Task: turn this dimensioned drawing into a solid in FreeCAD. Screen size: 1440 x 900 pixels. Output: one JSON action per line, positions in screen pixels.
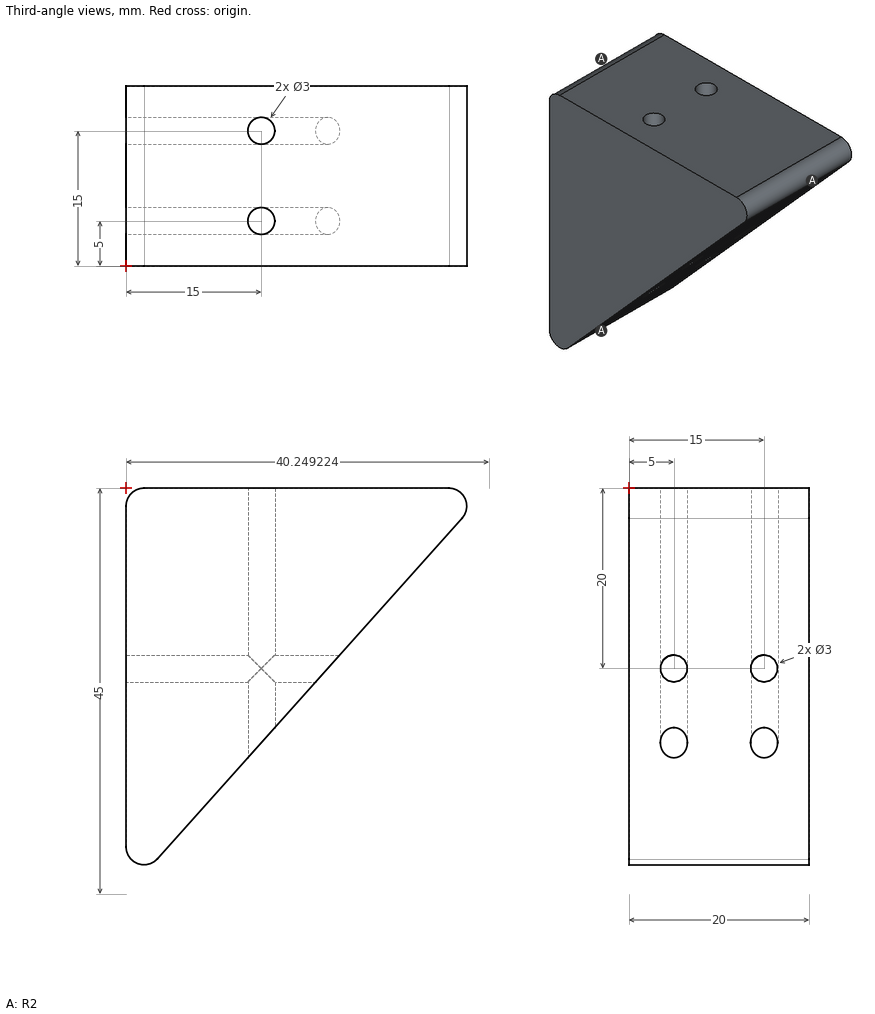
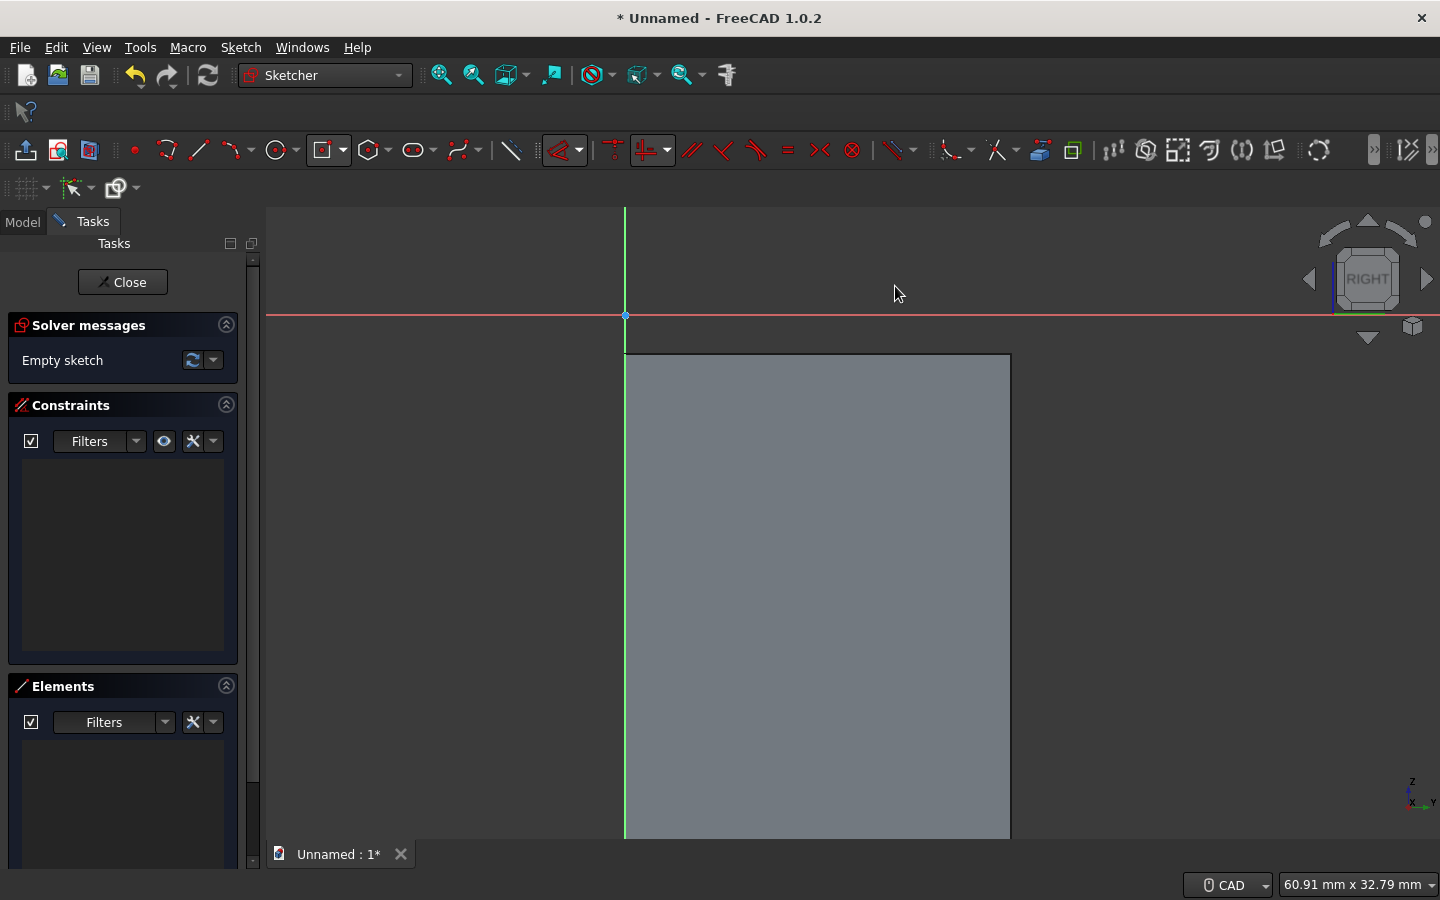
{"action": "key", "text": "g c"}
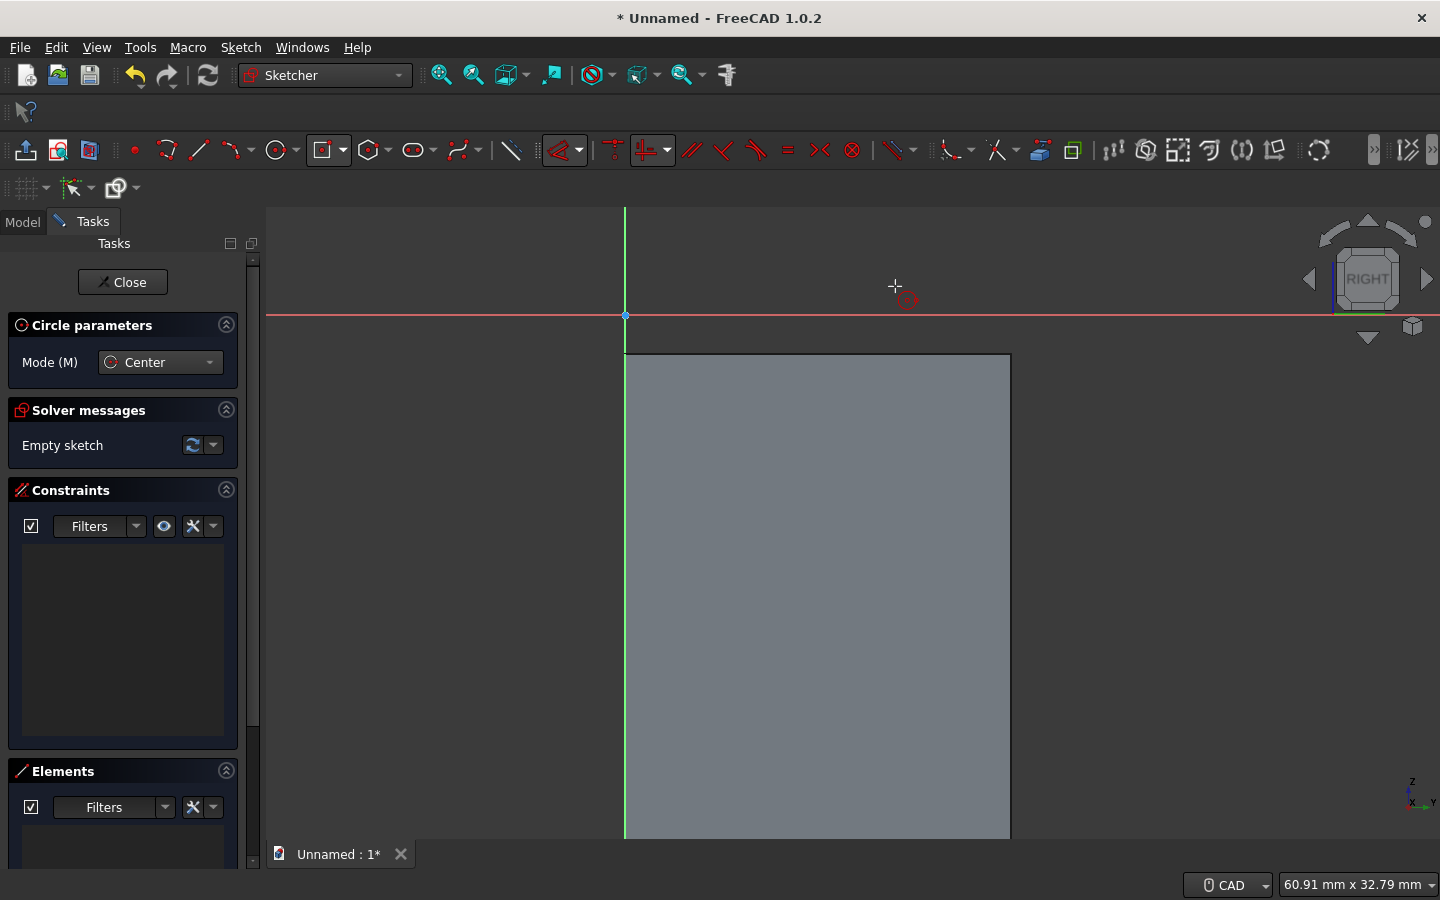
{"action": "left_click", "coordinate": [914, 701]}
{"action": "mouse_move", "coordinate": [935, 680]}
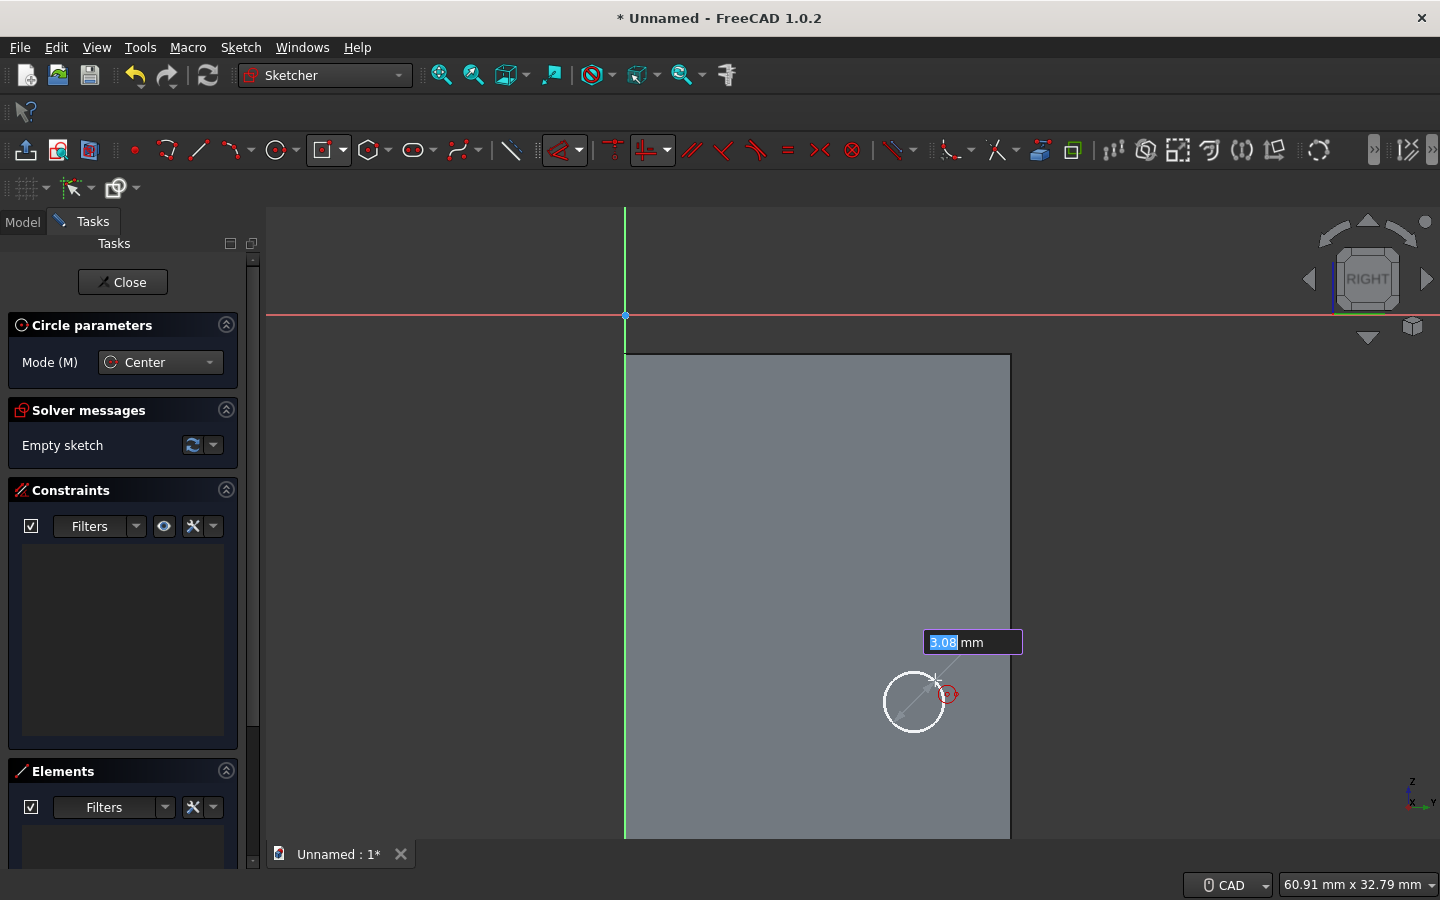
{"action": "type", "text": "3"}
{"action": "key", "text": "Return"}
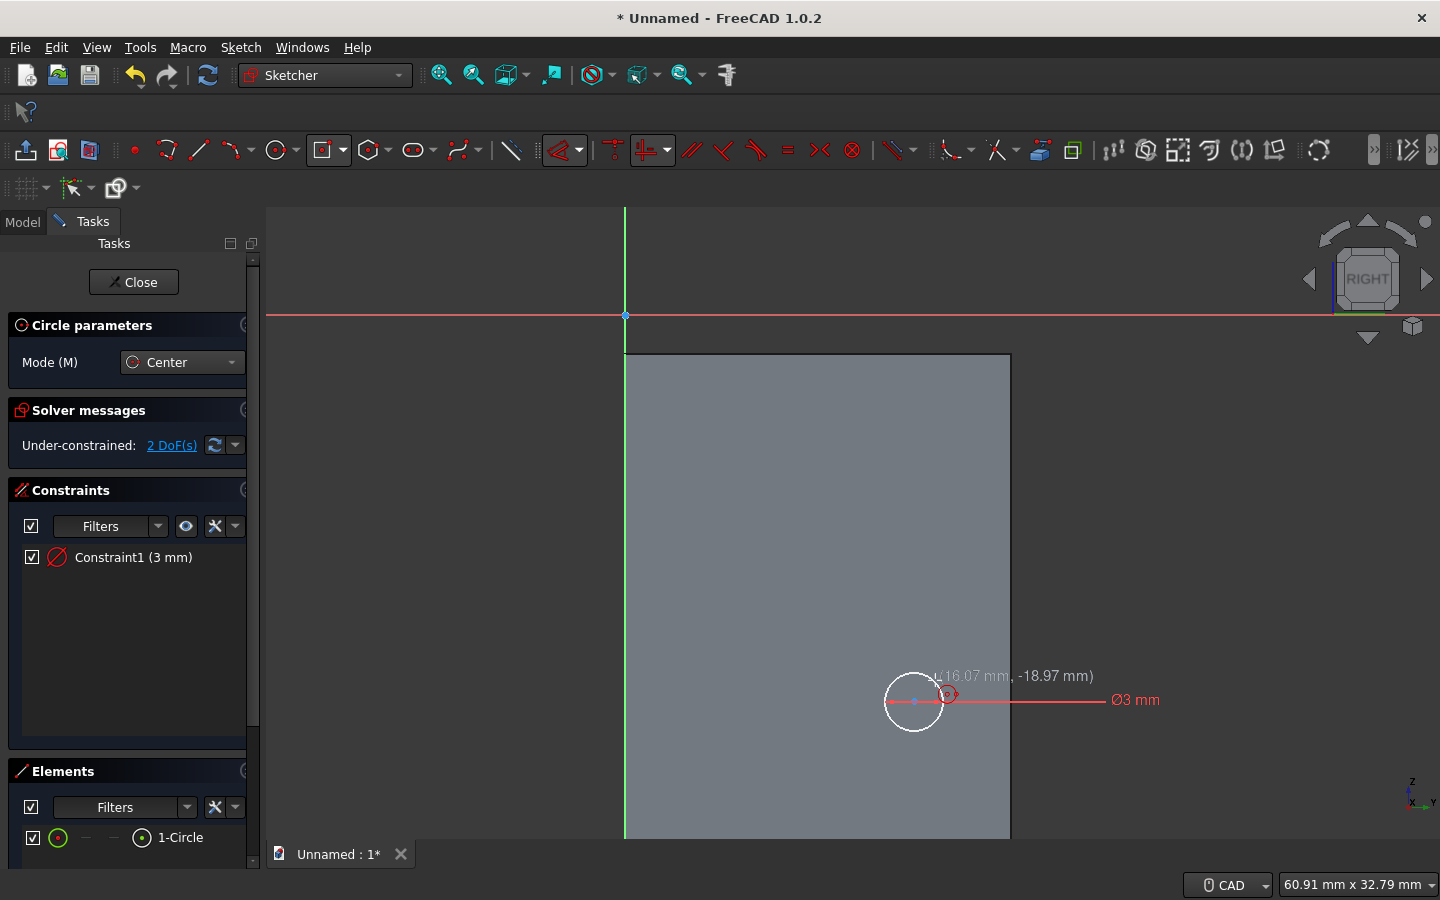
{"action": "left_click", "coordinate": [722, 701]}
{"action": "mouse_move", "coordinate": [742, 680]}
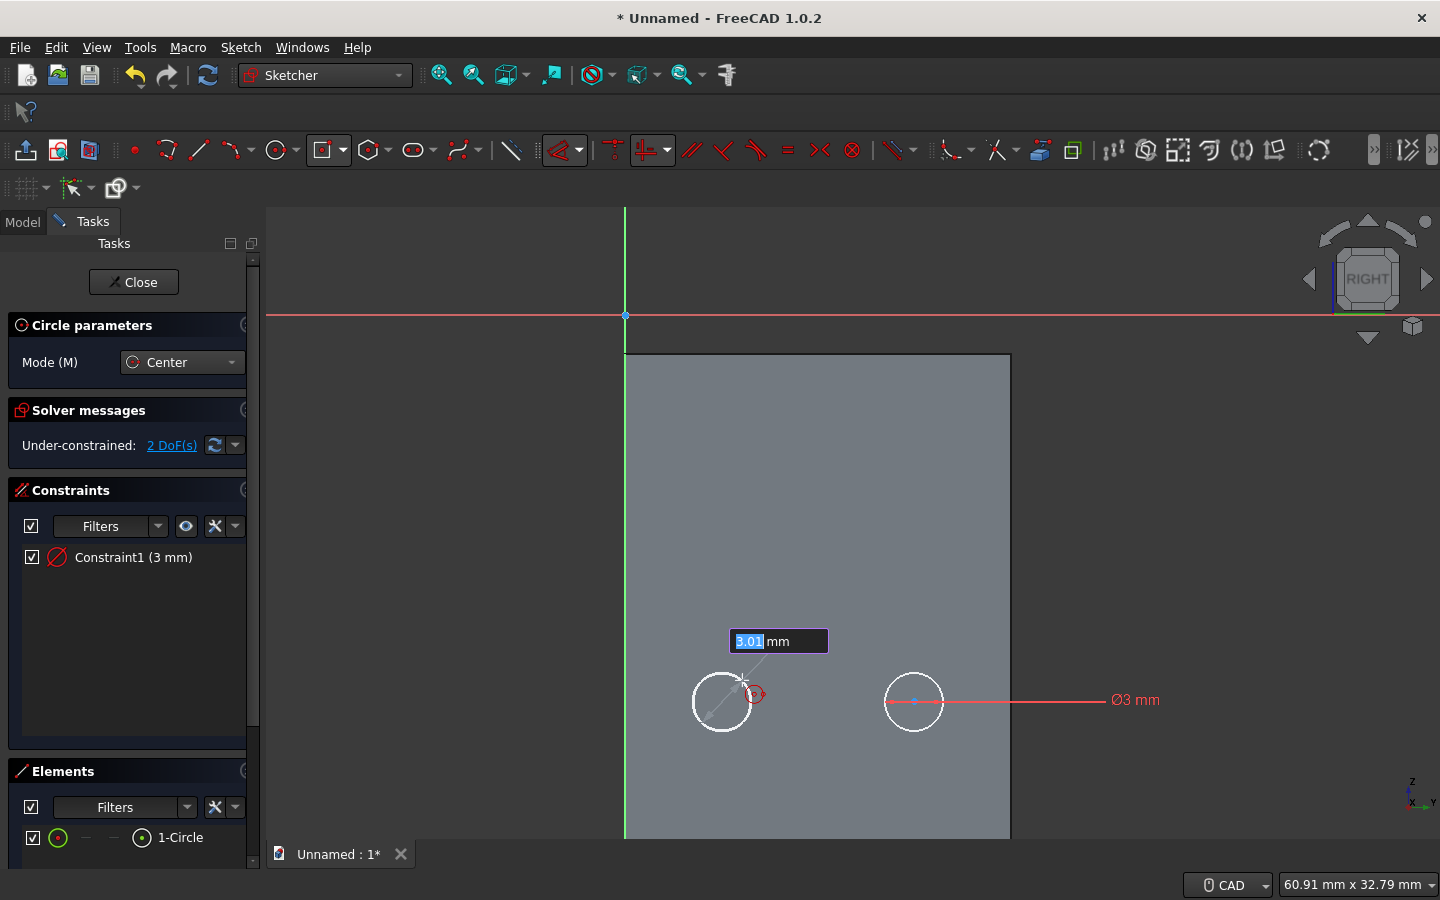
{"action": "type", "text": "3"}
{"action": "key", "text": "Return"}
{"action": "key", "text": "Escape"}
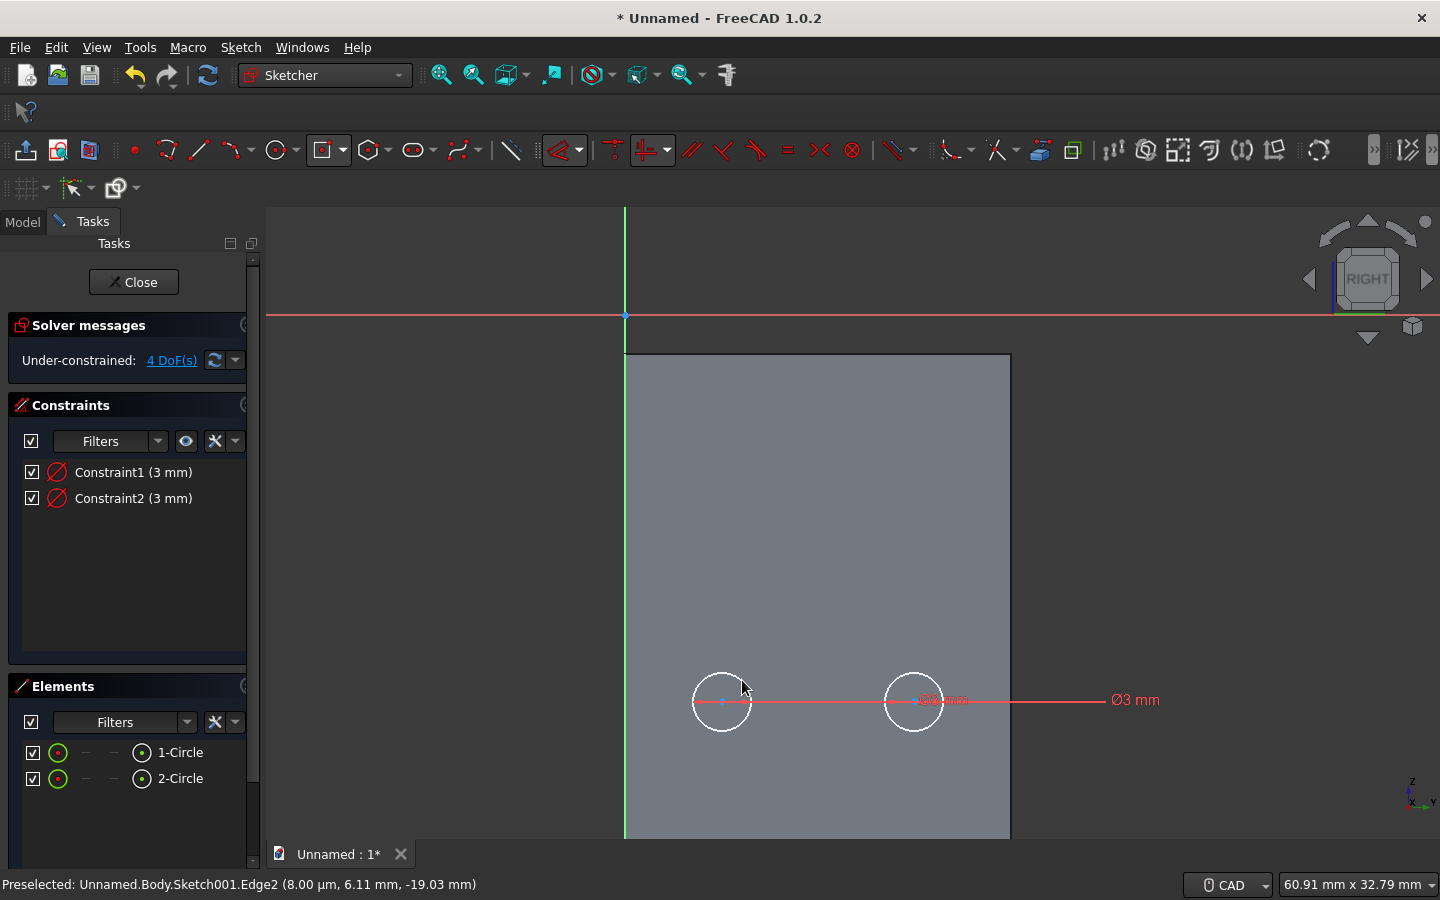
{"action": "left_click", "coordinate": [914, 702]}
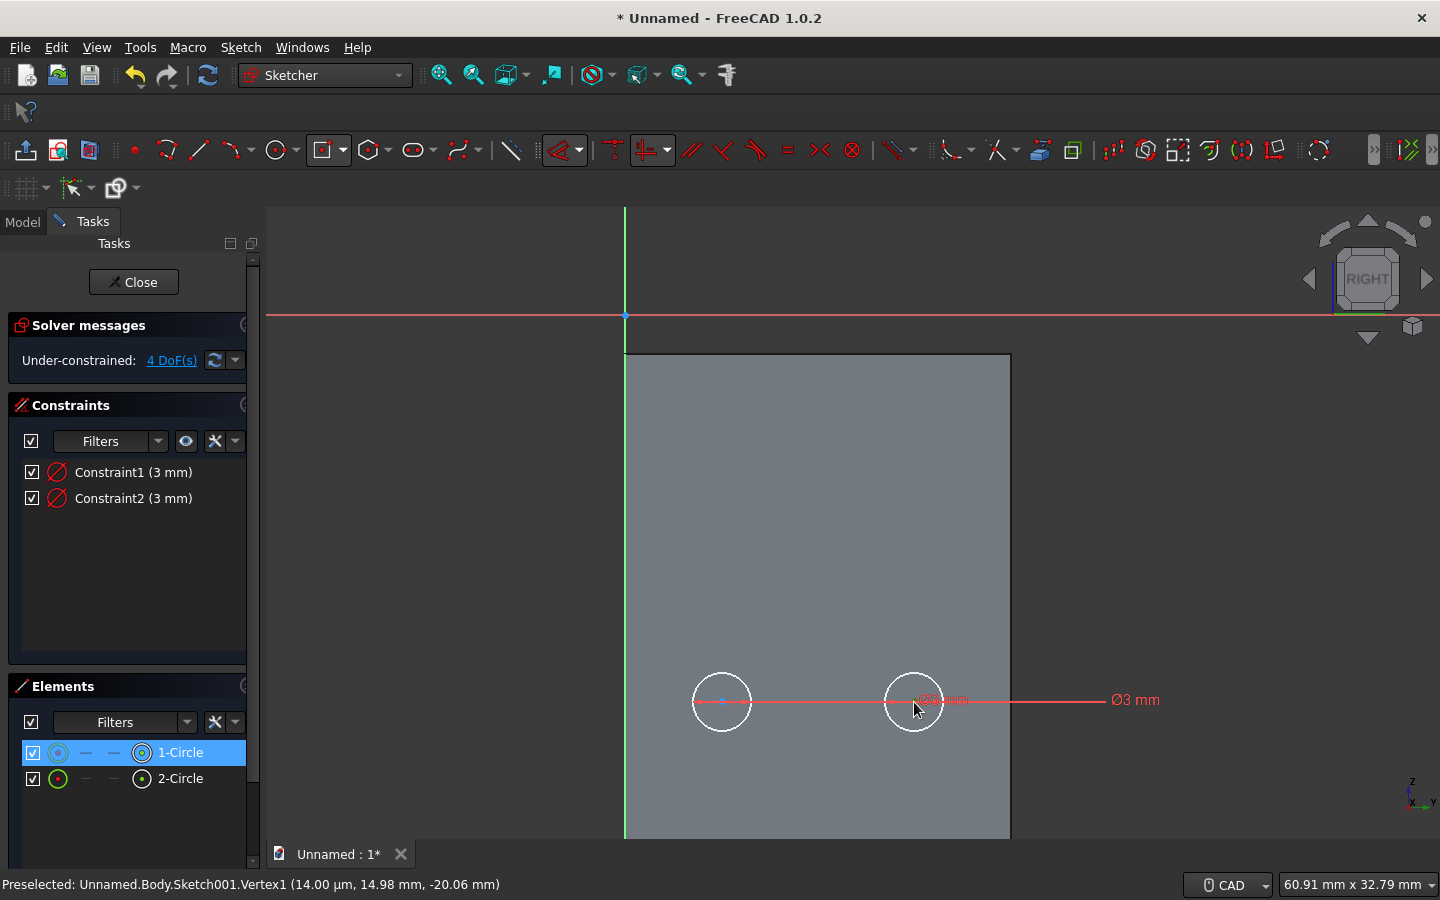
{"action": "left_click", "coordinate": [722, 702]}